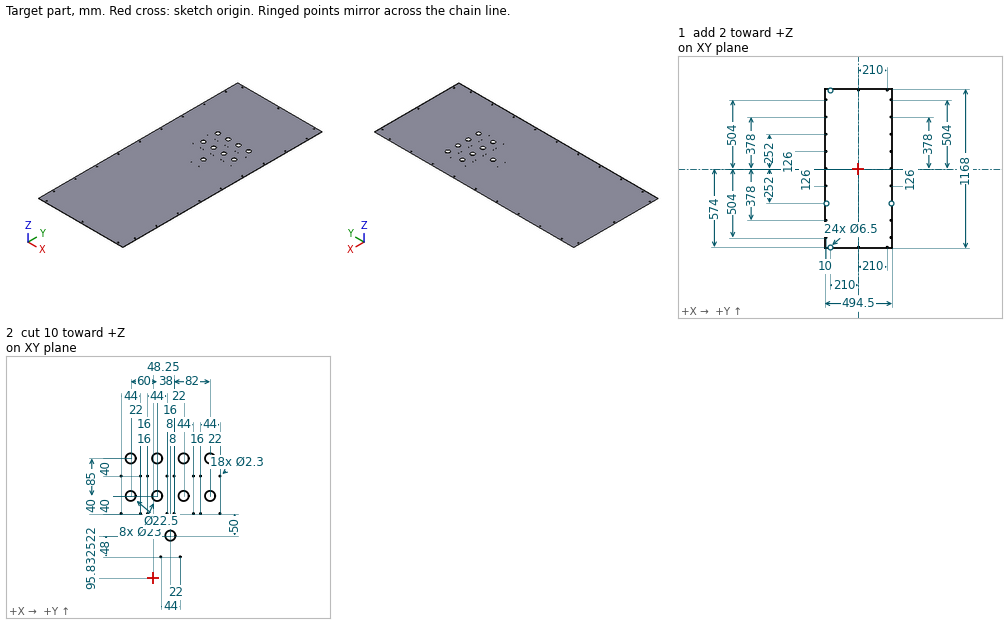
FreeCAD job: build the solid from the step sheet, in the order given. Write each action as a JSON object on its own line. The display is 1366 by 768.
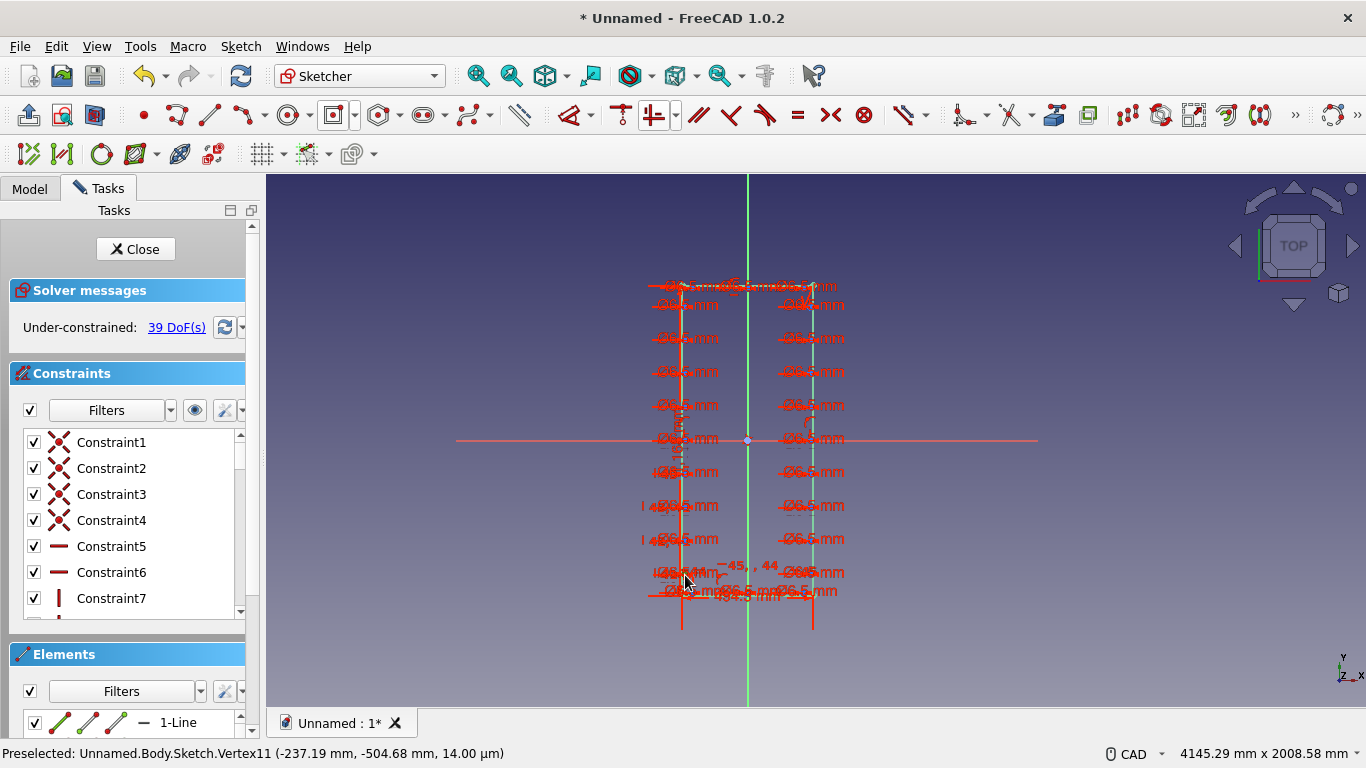
{"action": "scroll", "coordinate": [811, 574], "scroll_direction": "up", "scroll_amount": 4}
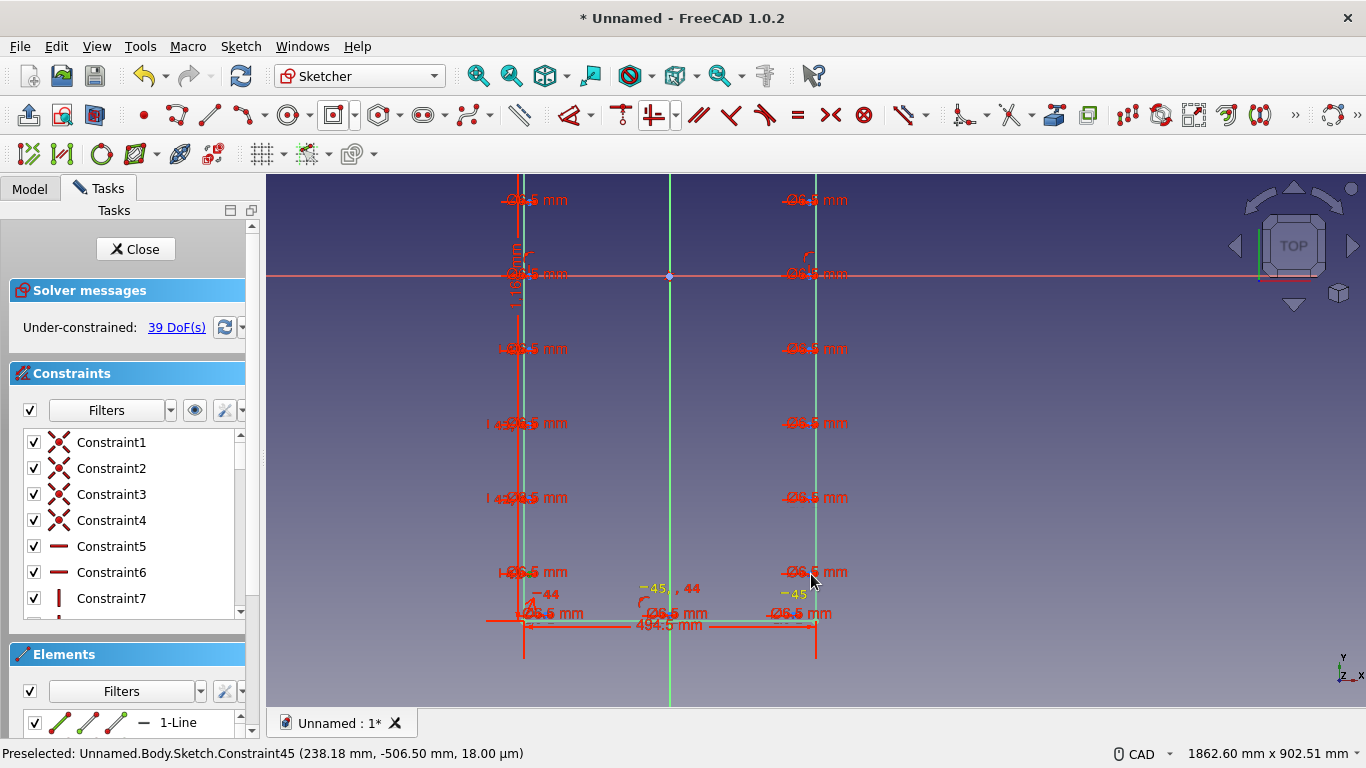
{"action": "left_click", "coordinate": [810, 574]}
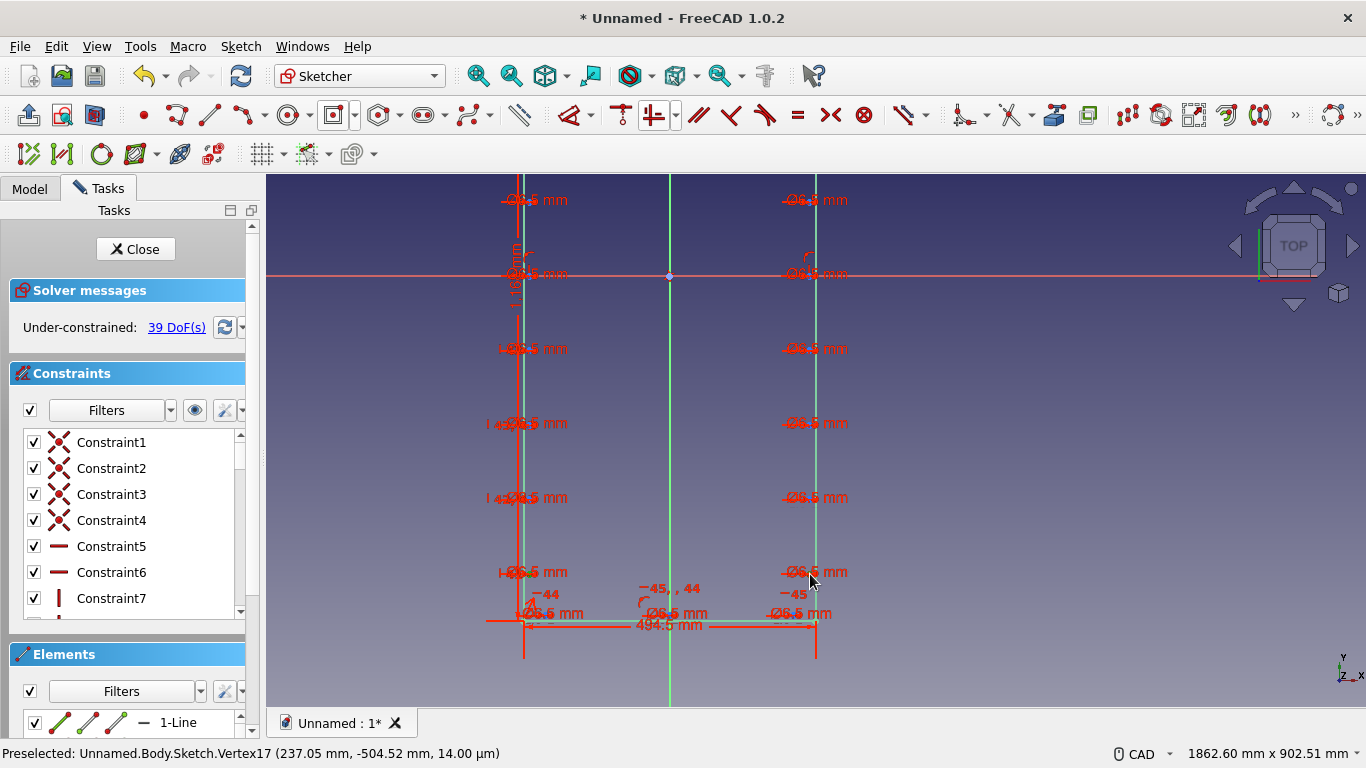
{"action": "left_click", "coordinate": [676, 116]}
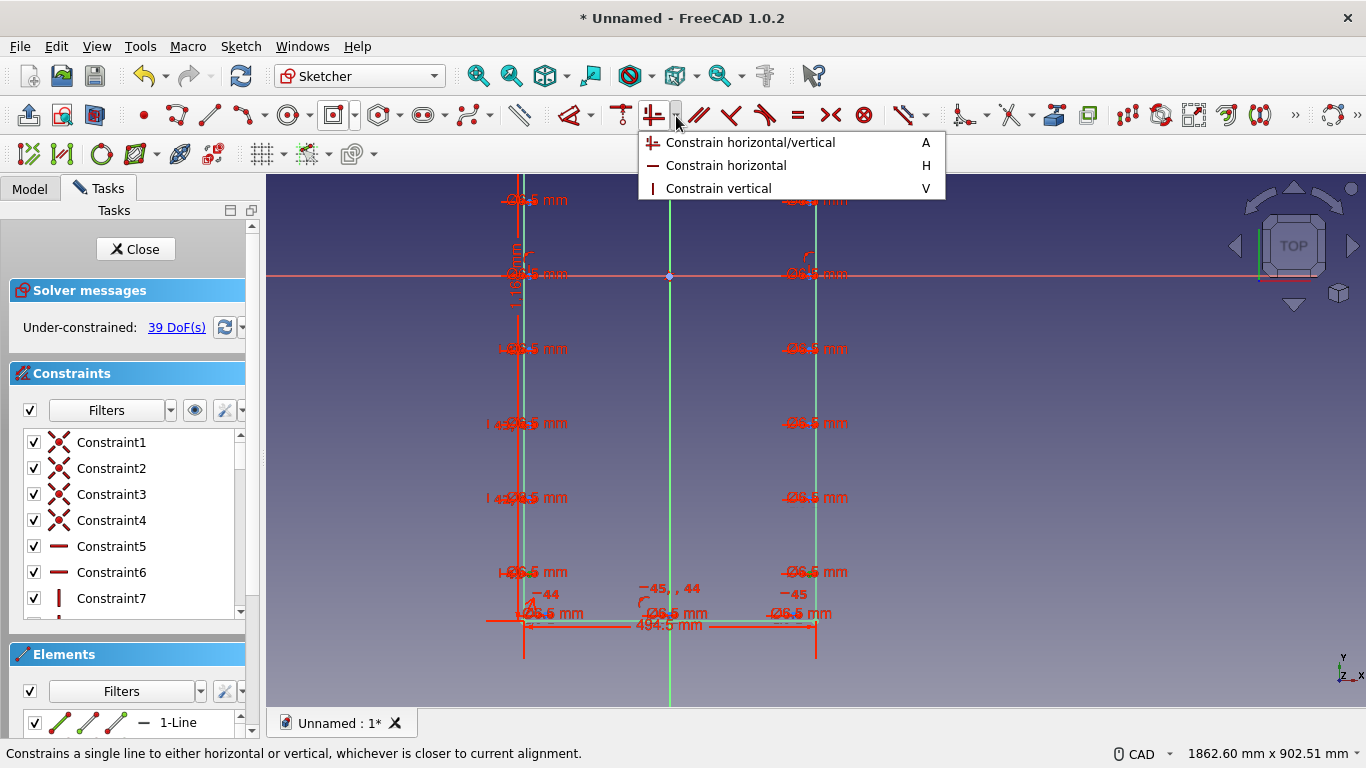
{"action": "left_click", "coordinate": [792, 166]}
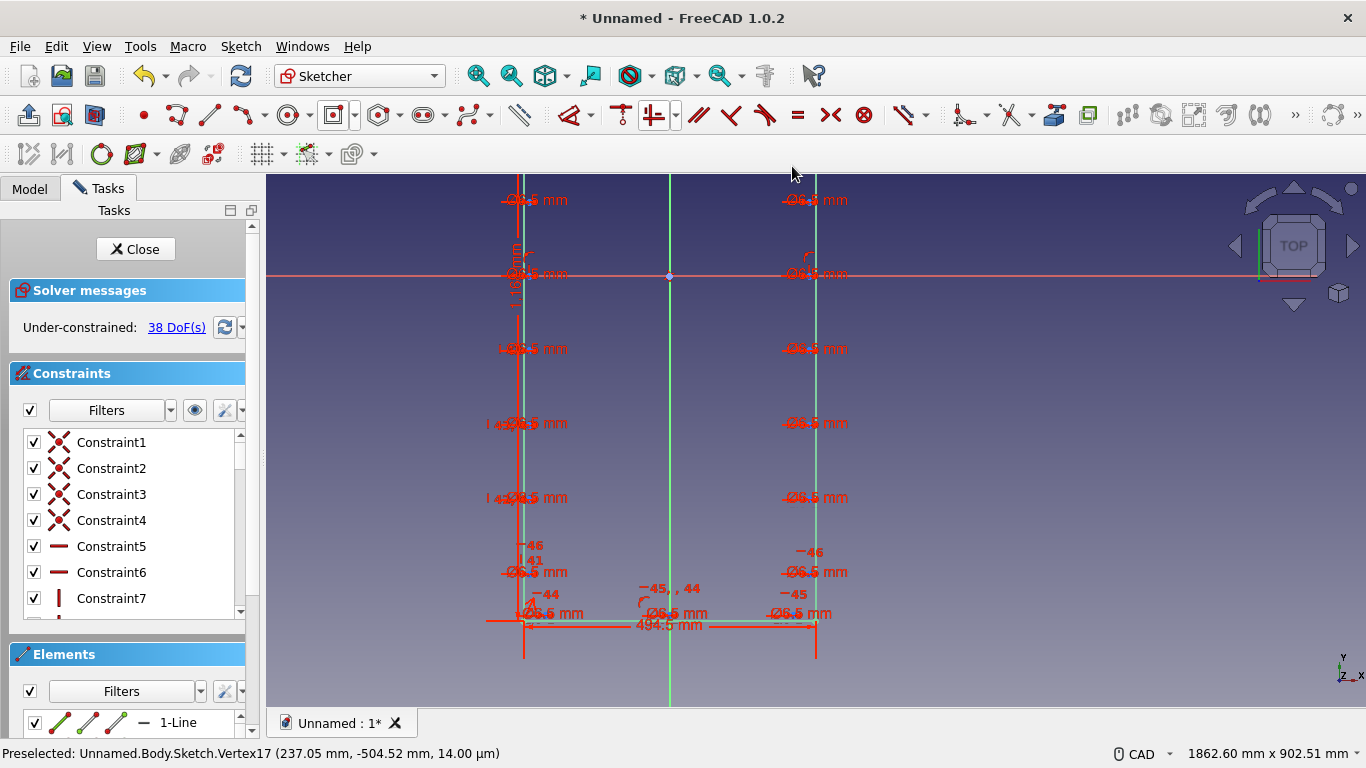
{"action": "left_click", "coordinate": [810, 574]}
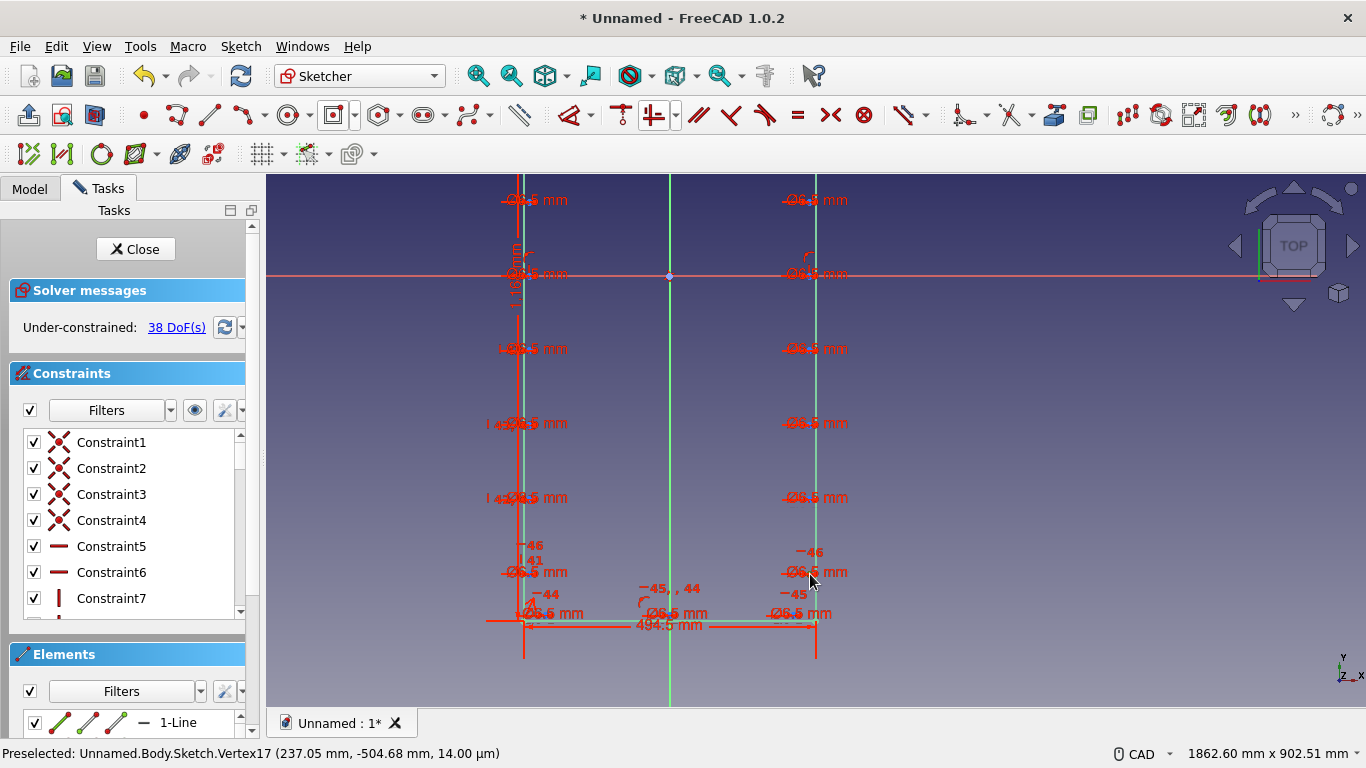
{"action": "left_click", "coordinate": [810, 500]}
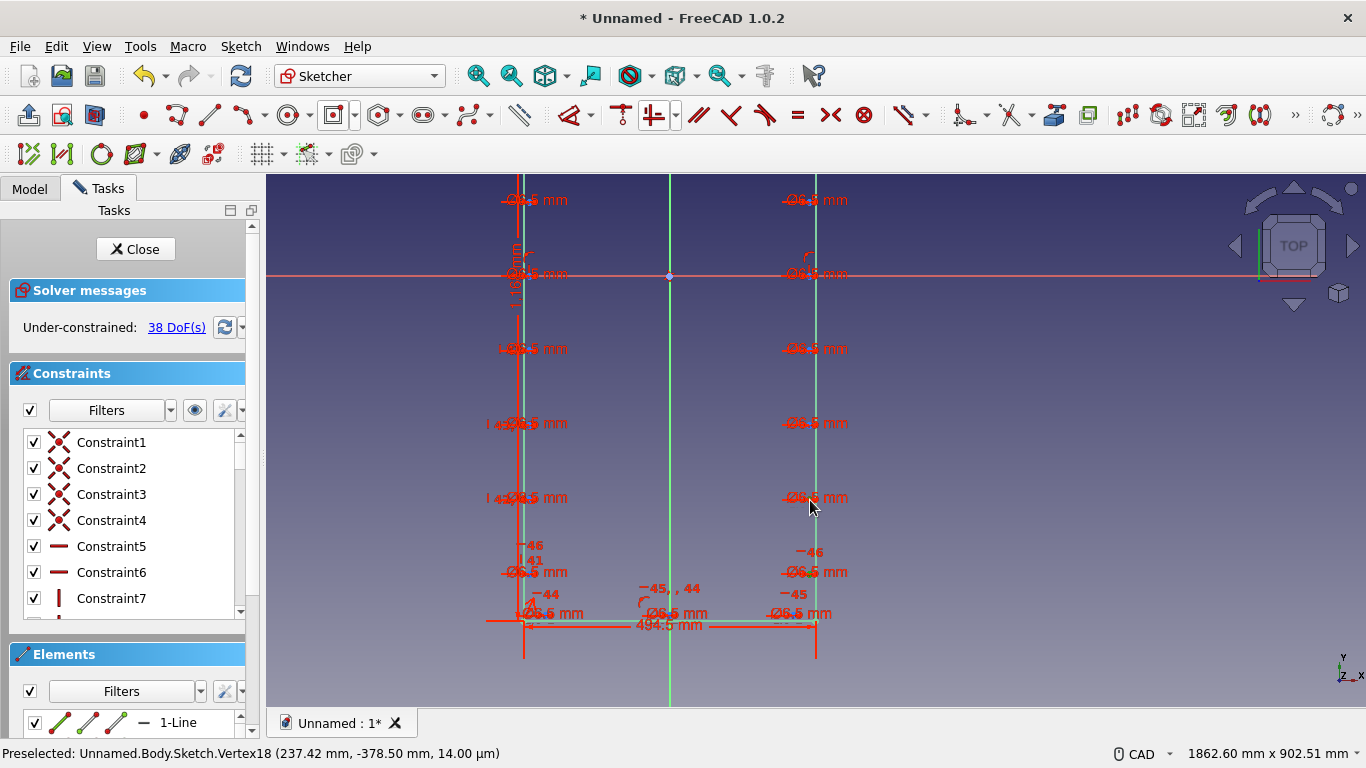
{"action": "key", "text": "v"}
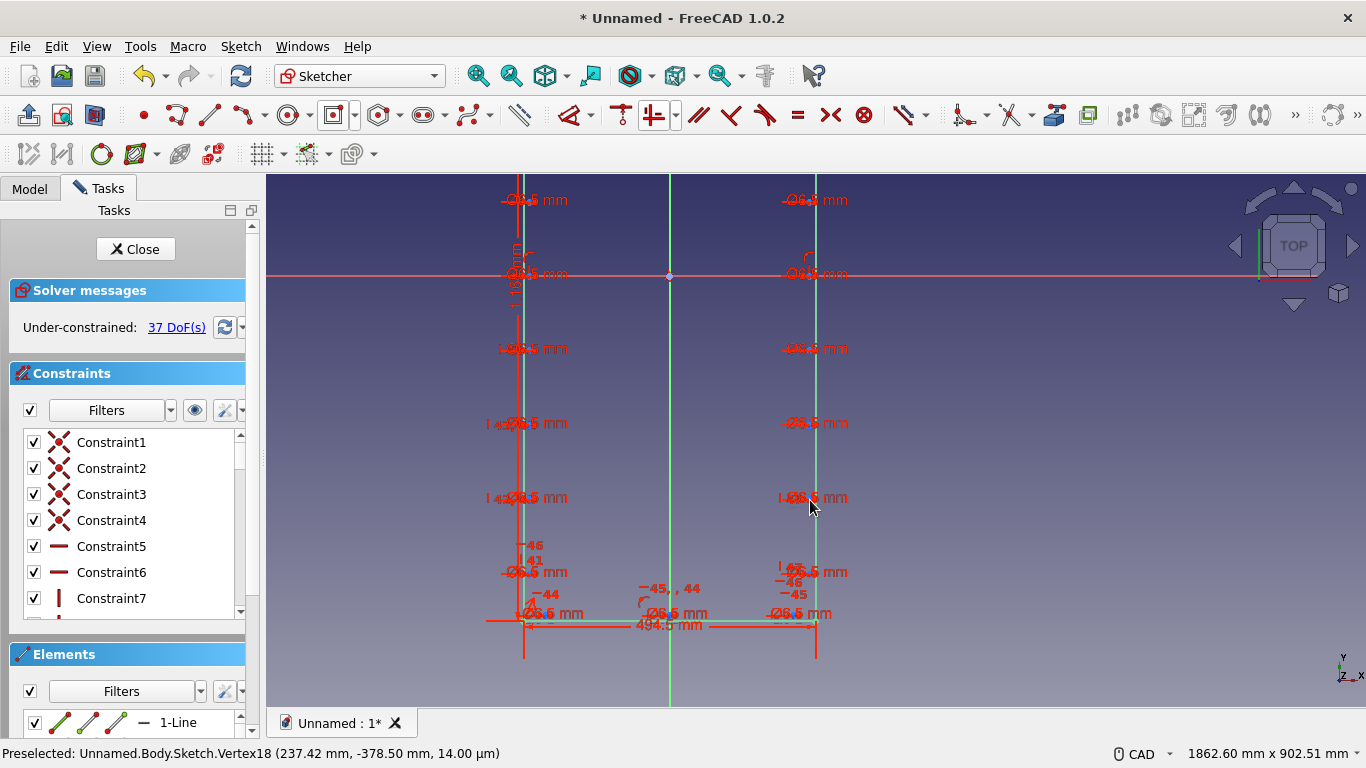
{"action": "left_click", "coordinate": [530, 500]}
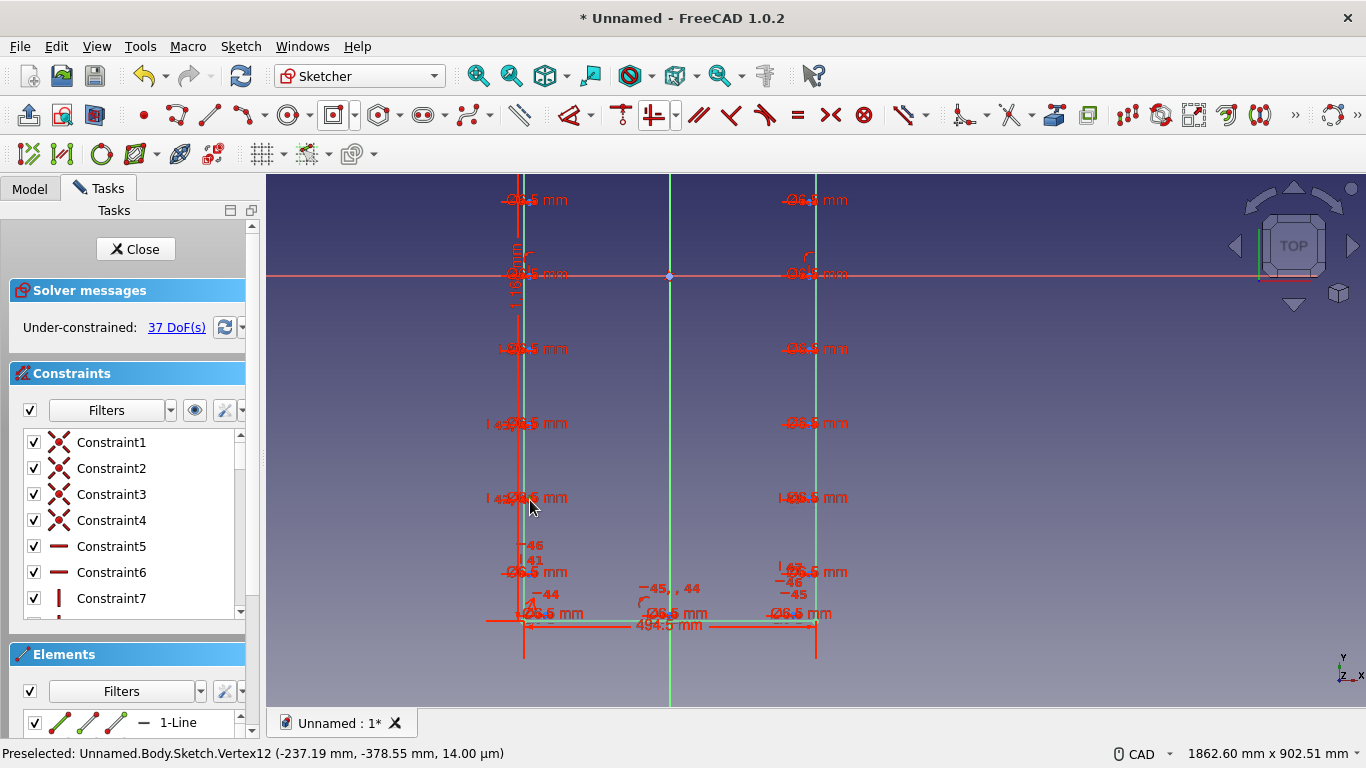
{"action": "left_click", "coordinate": [810, 500]}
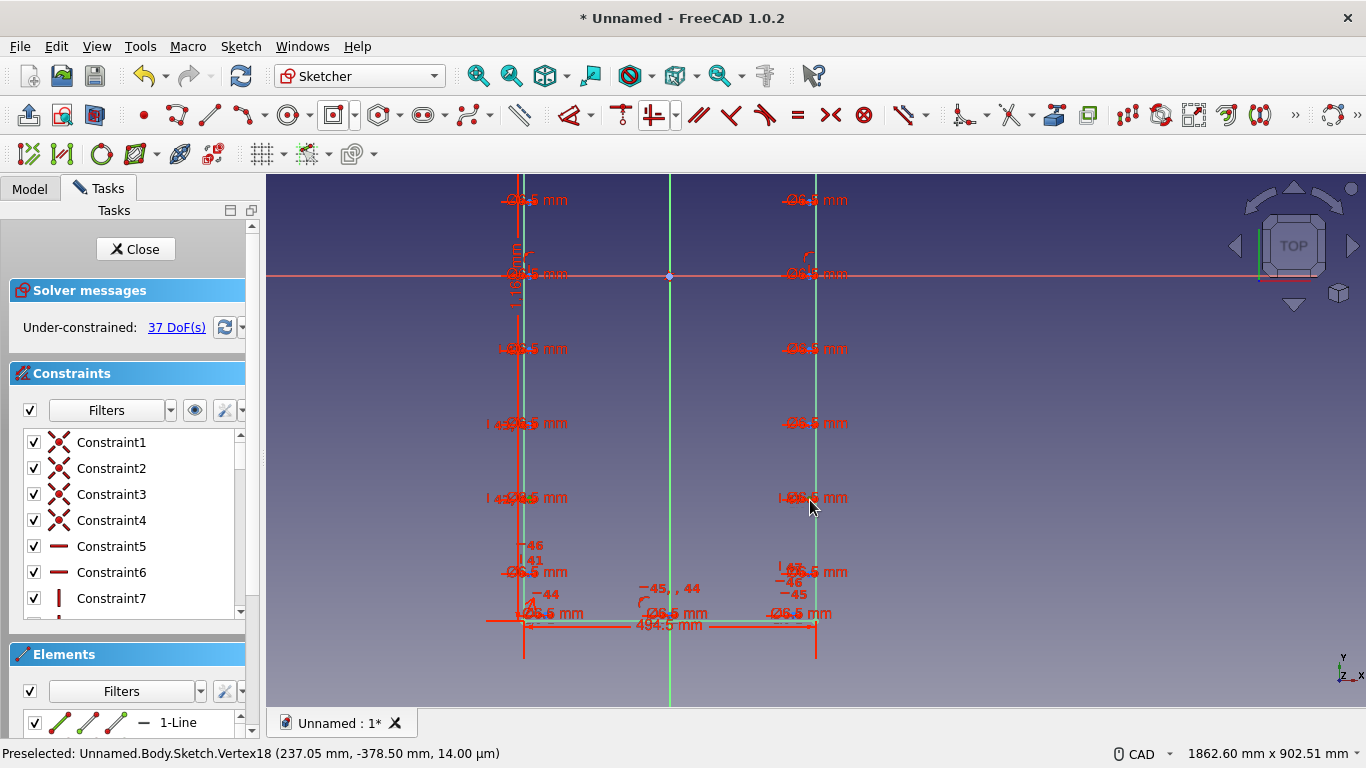
{"action": "left_click", "coordinate": [676, 116]}